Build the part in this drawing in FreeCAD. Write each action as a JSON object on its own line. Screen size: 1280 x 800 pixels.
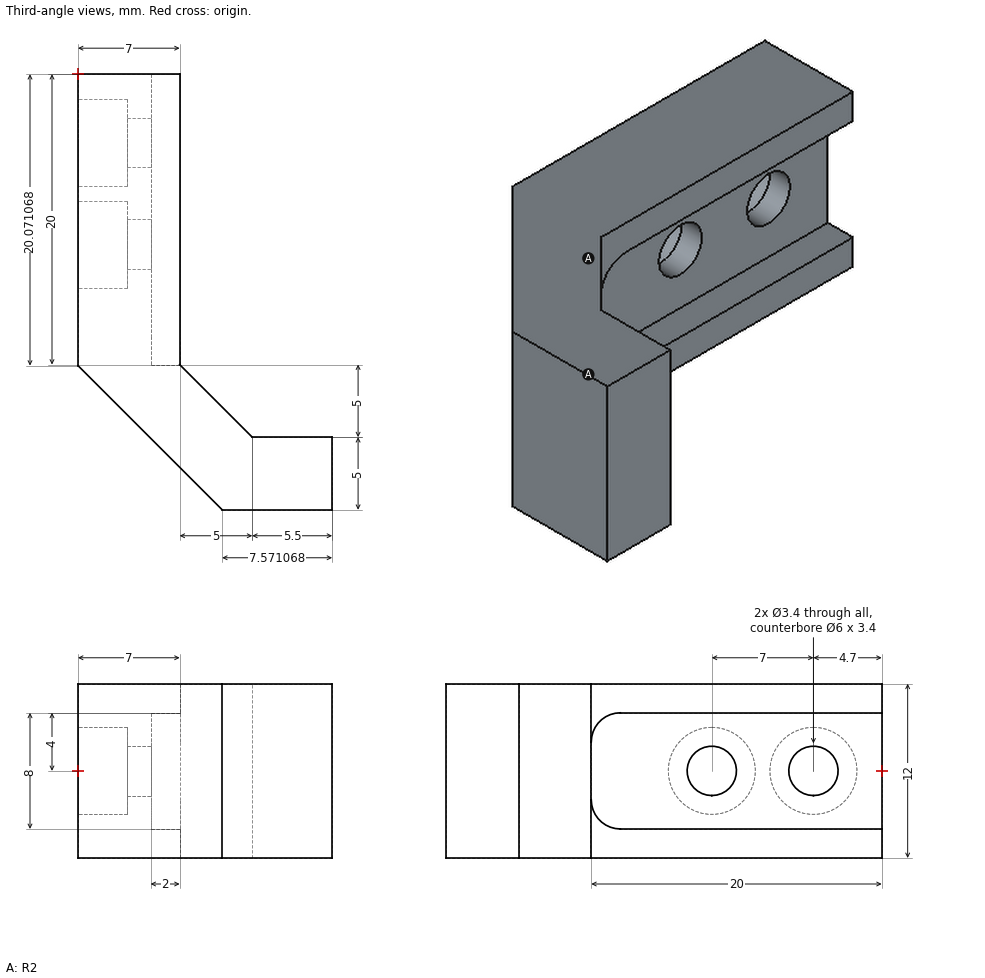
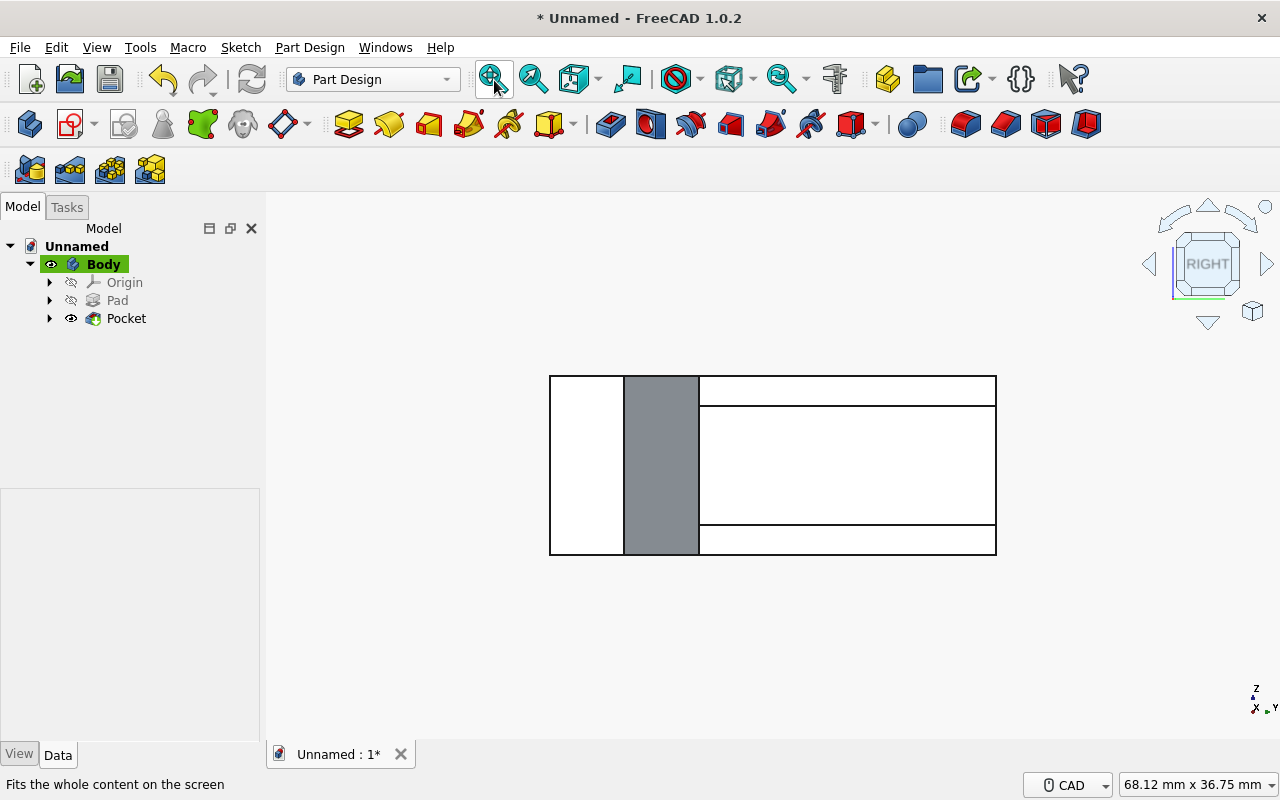
{"action": "left_click", "coordinate": [494, 80]}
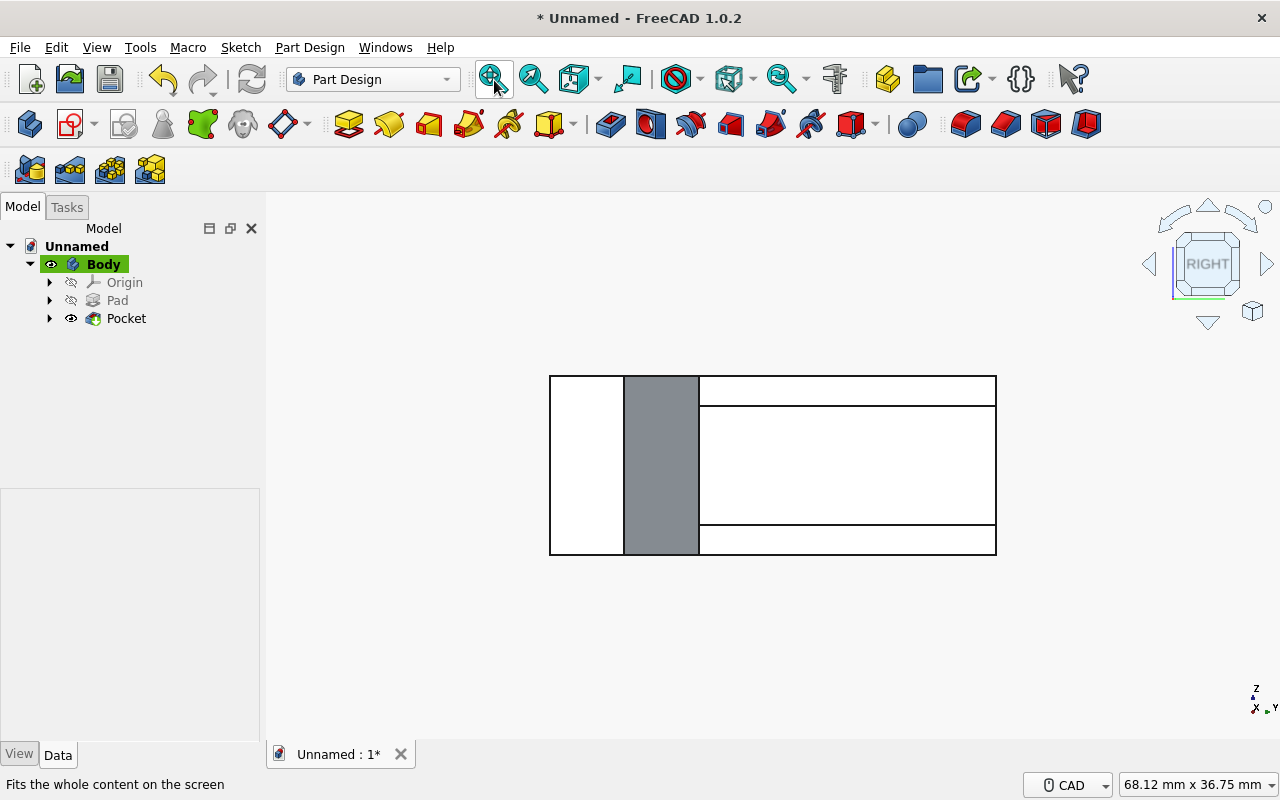
{"action": "key", "text": "5"}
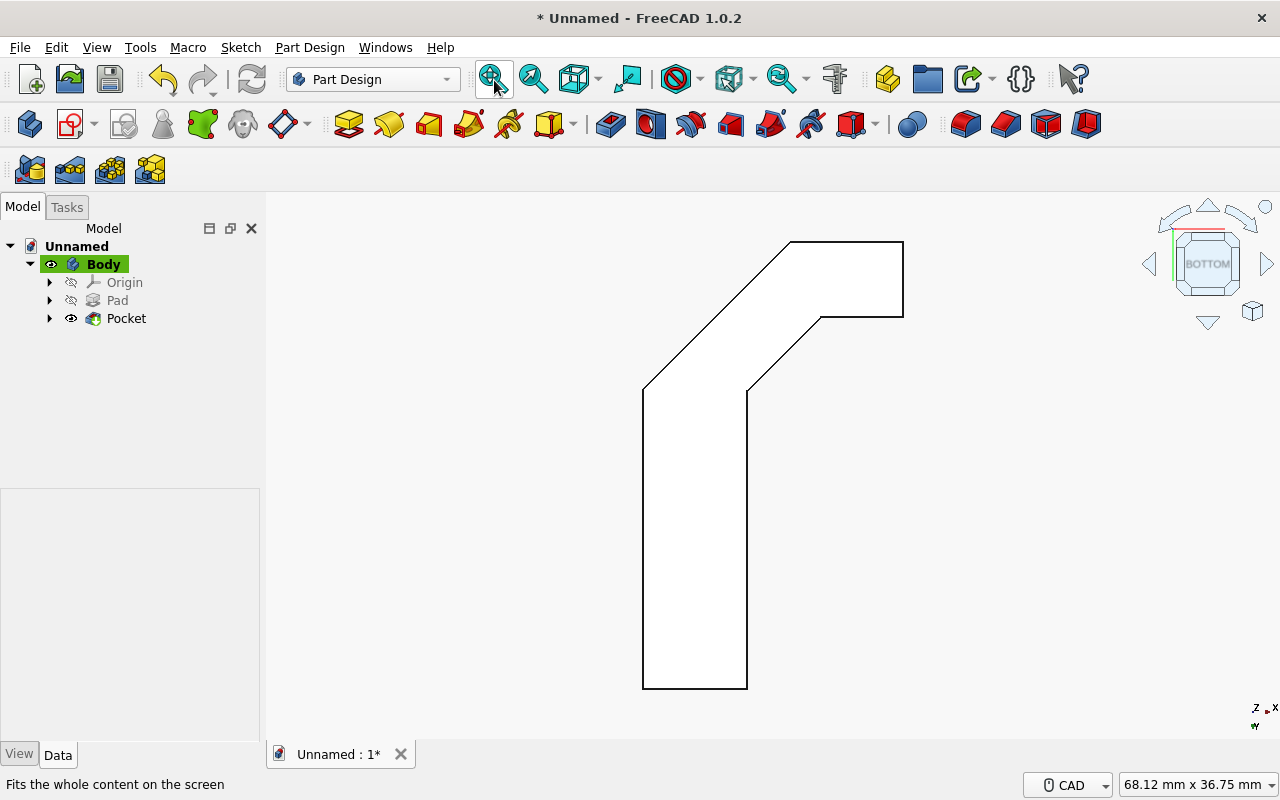
{"action": "key", "text": "4"}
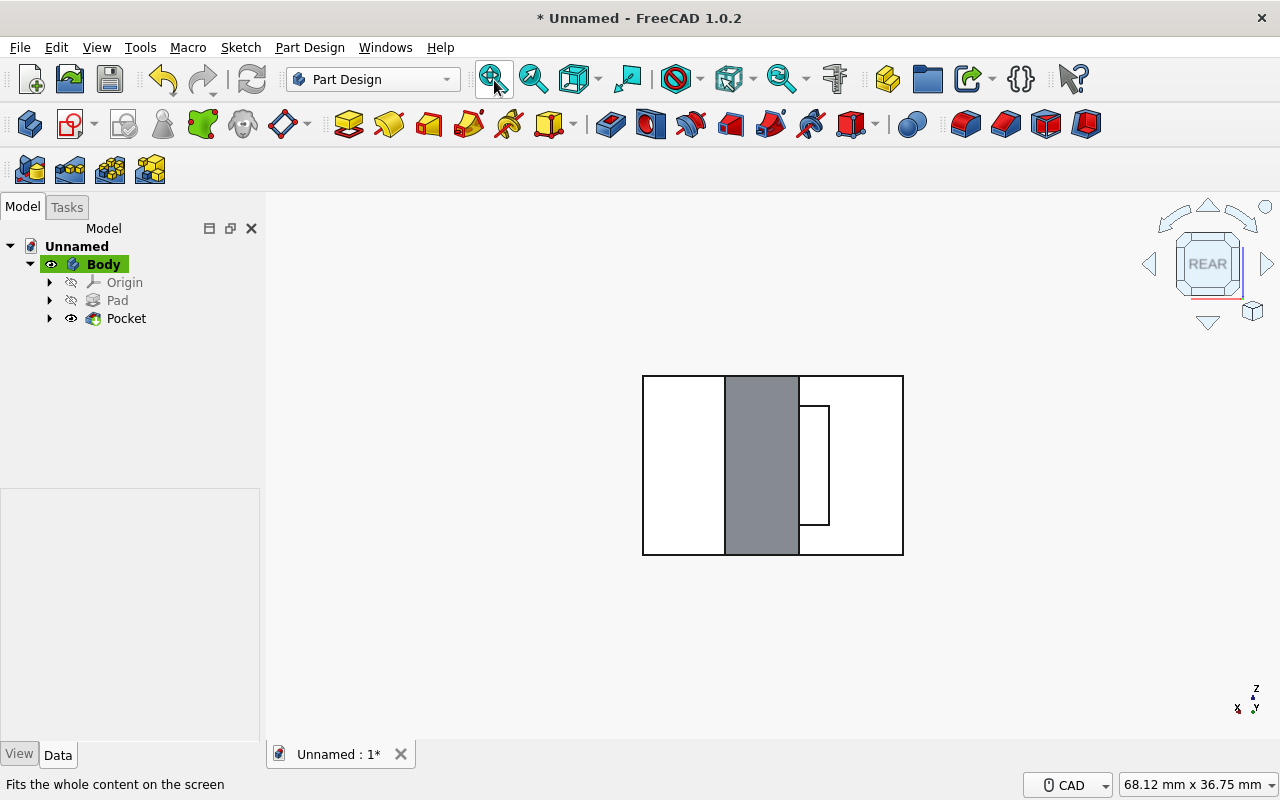
{"action": "left_click", "coordinate": [494, 80]}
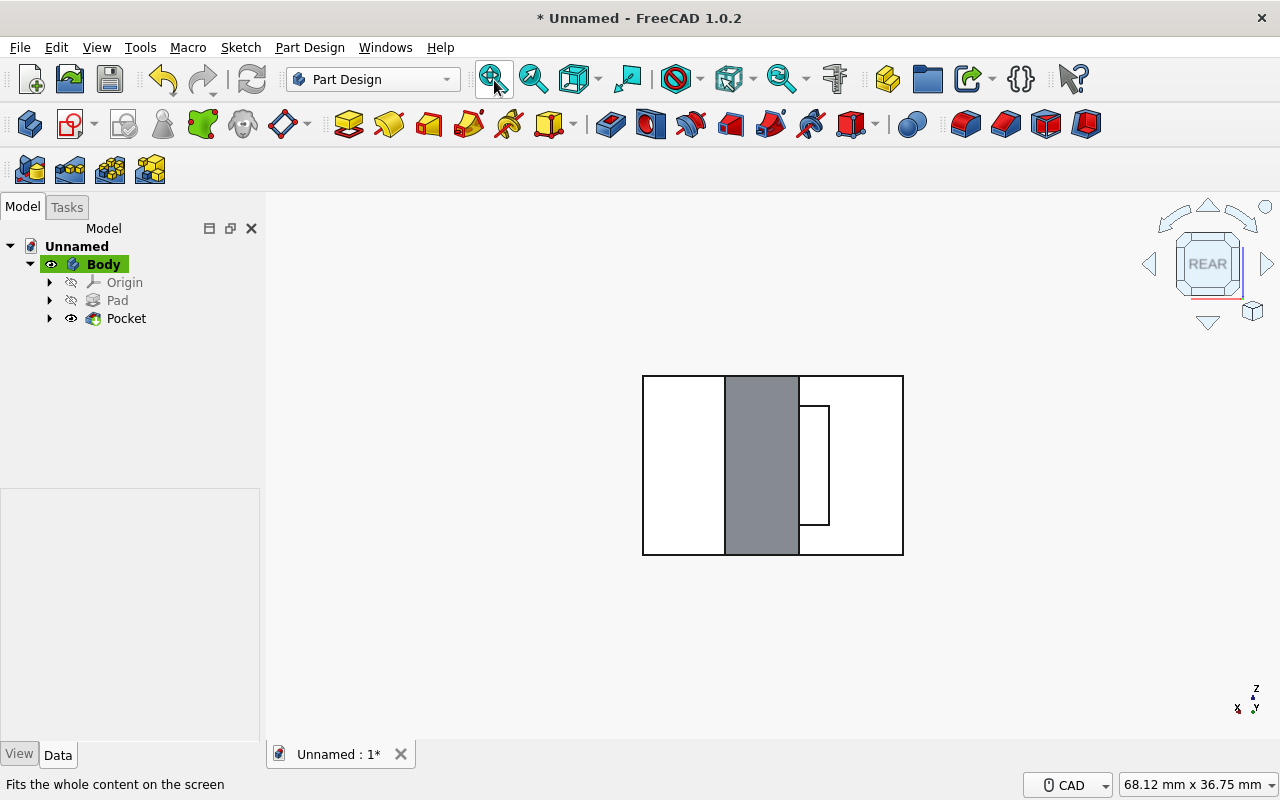
{"action": "key", "text": "6"}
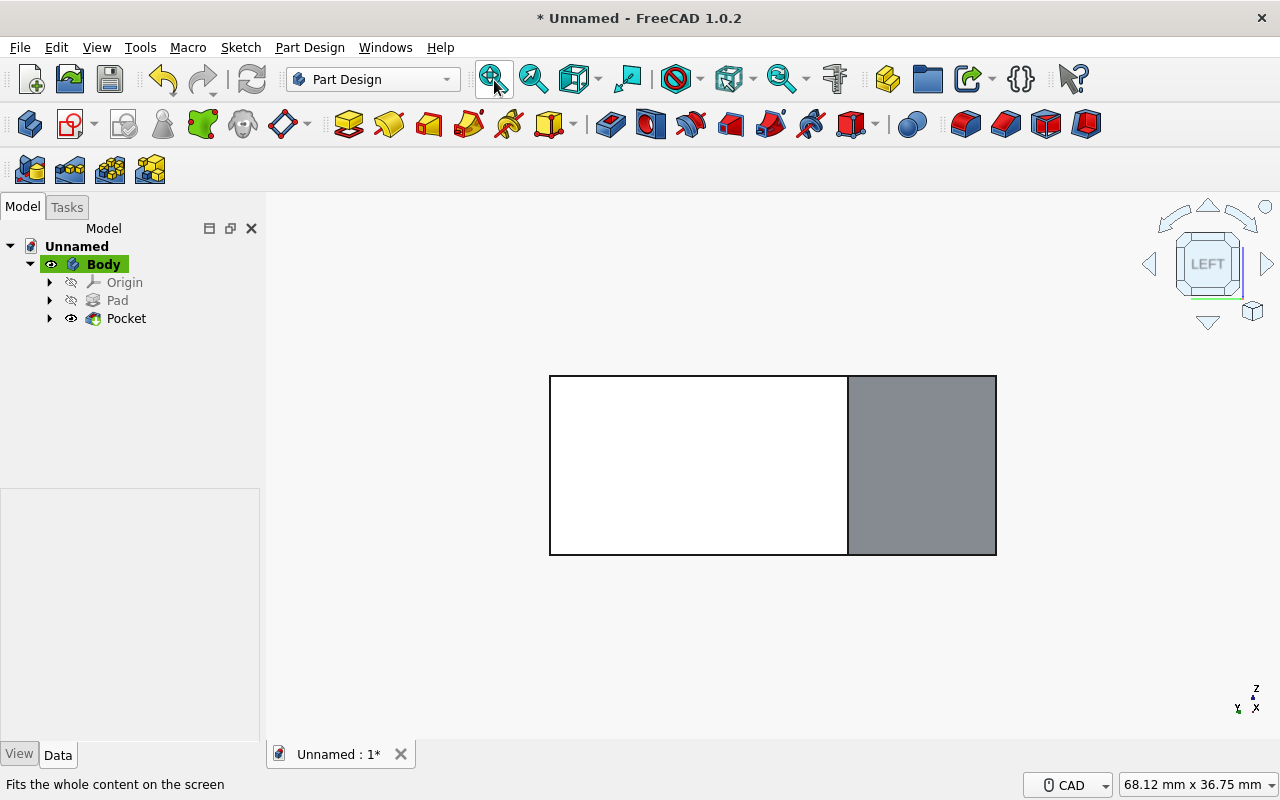
{"action": "left_click", "coordinate": [494, 80]}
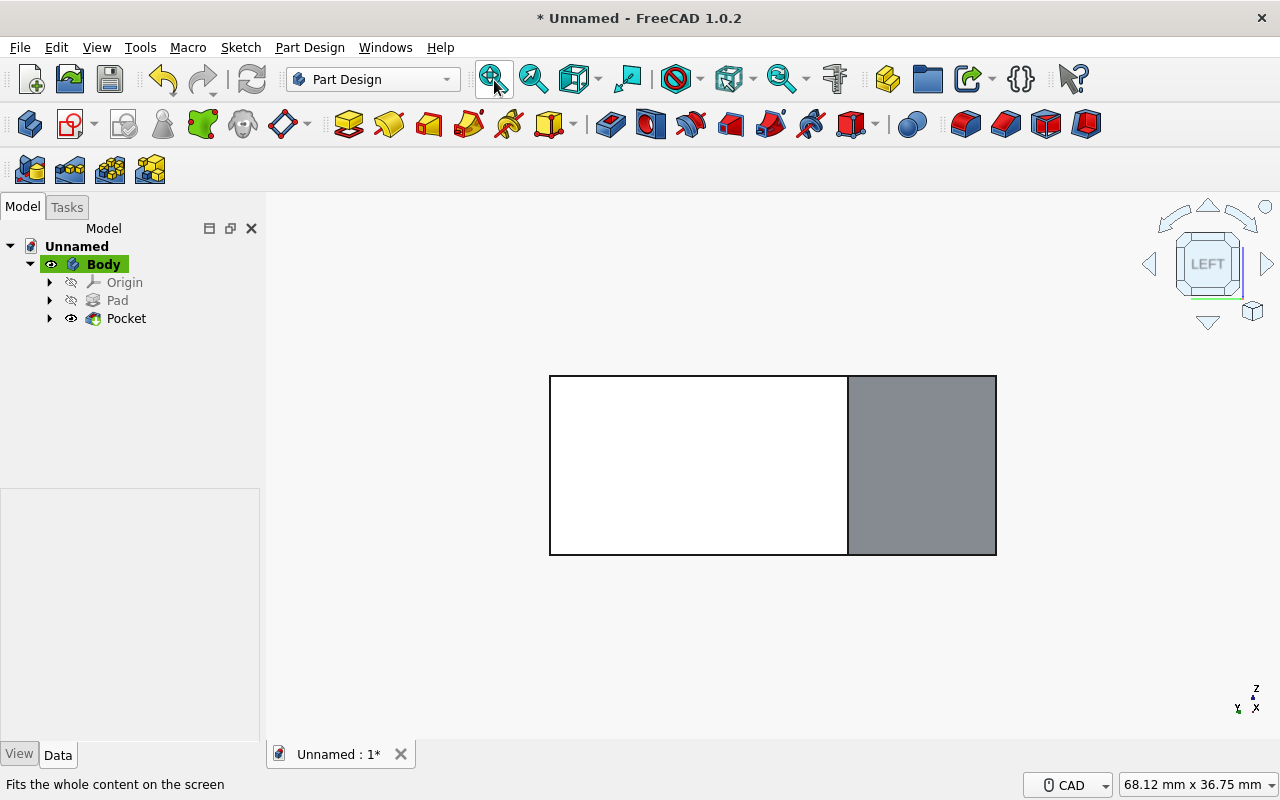
{"action": "key", "text": "v 3"}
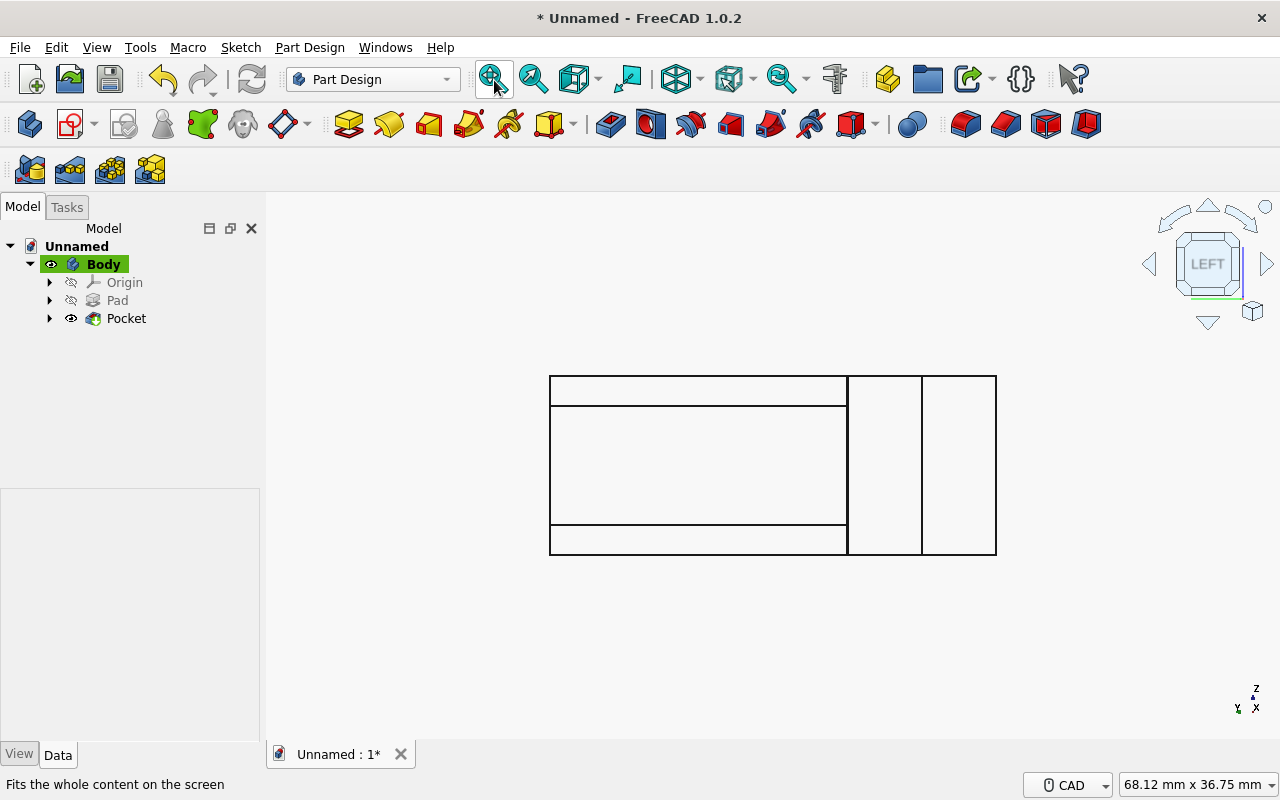
{"action": "key", "text": "0"}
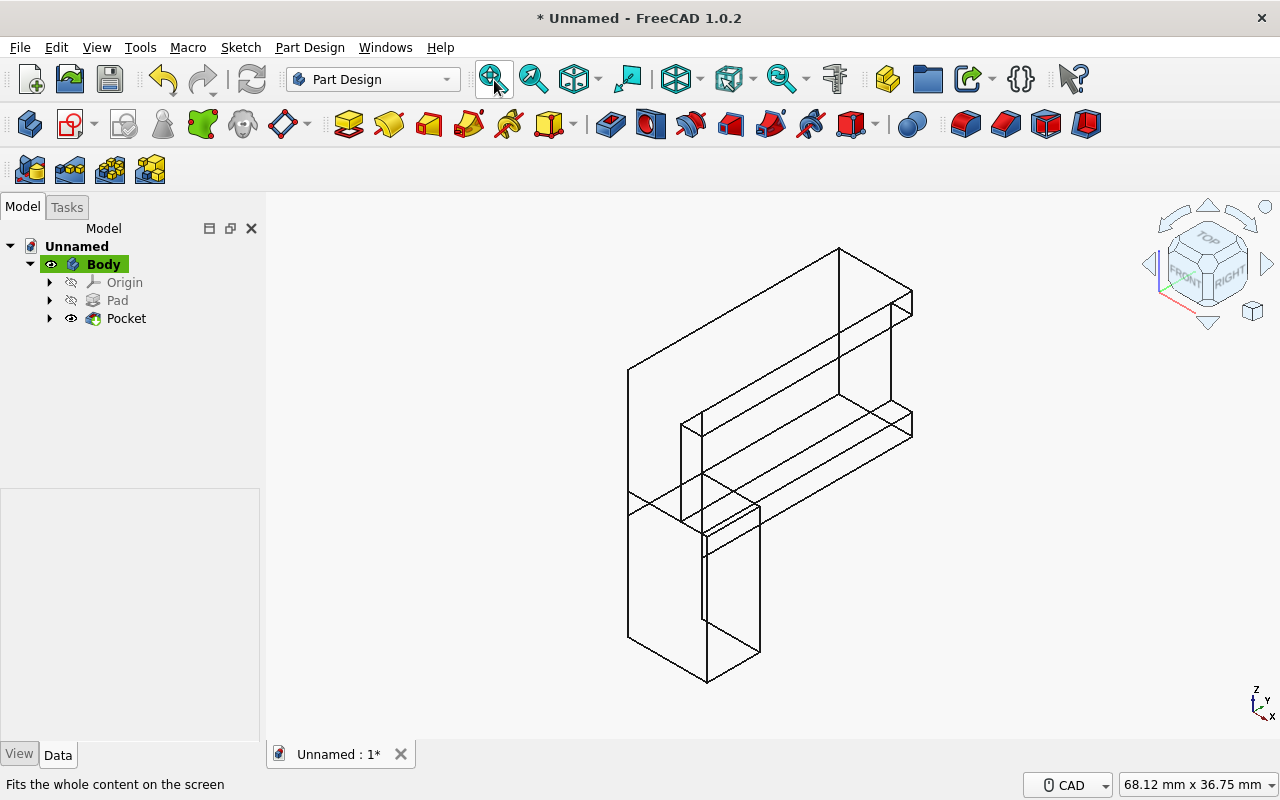
{"action": "left_click", "coordinate": [691, 430]}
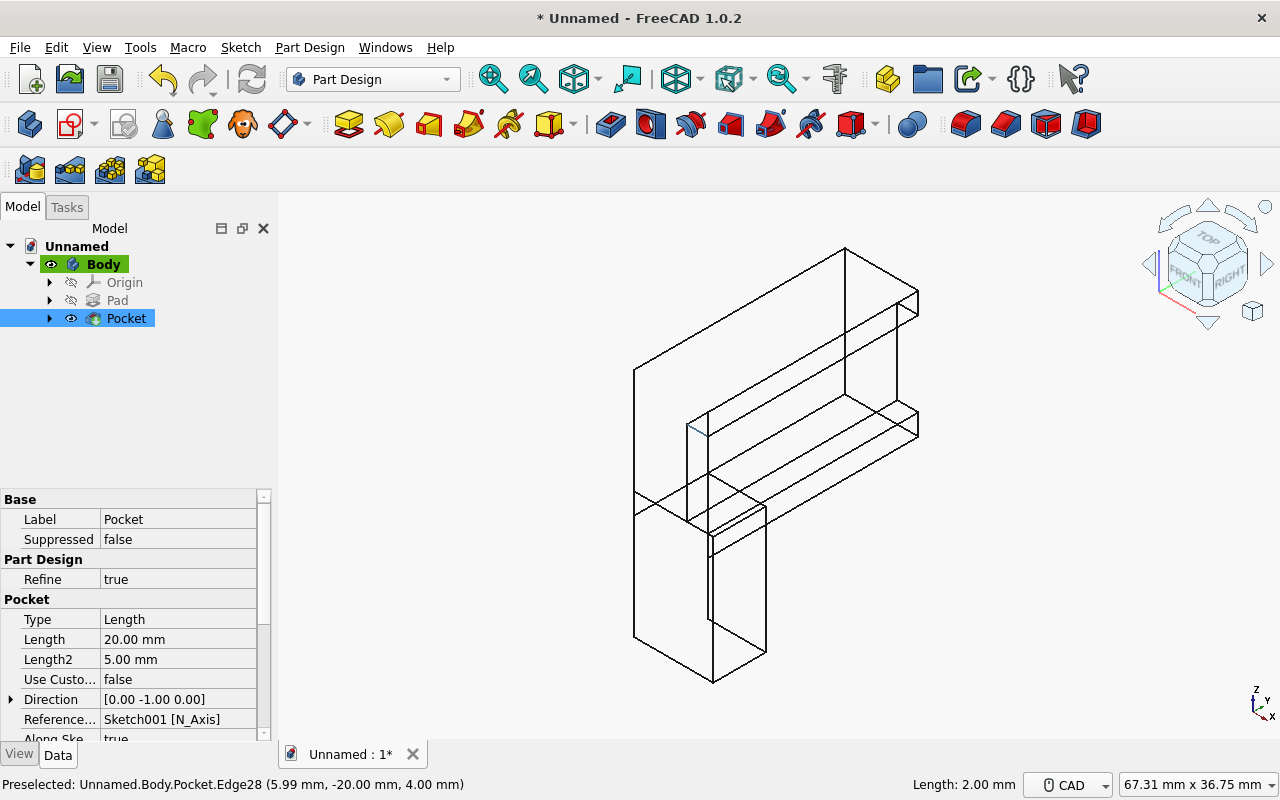
{"action": "key", "text": "2"}